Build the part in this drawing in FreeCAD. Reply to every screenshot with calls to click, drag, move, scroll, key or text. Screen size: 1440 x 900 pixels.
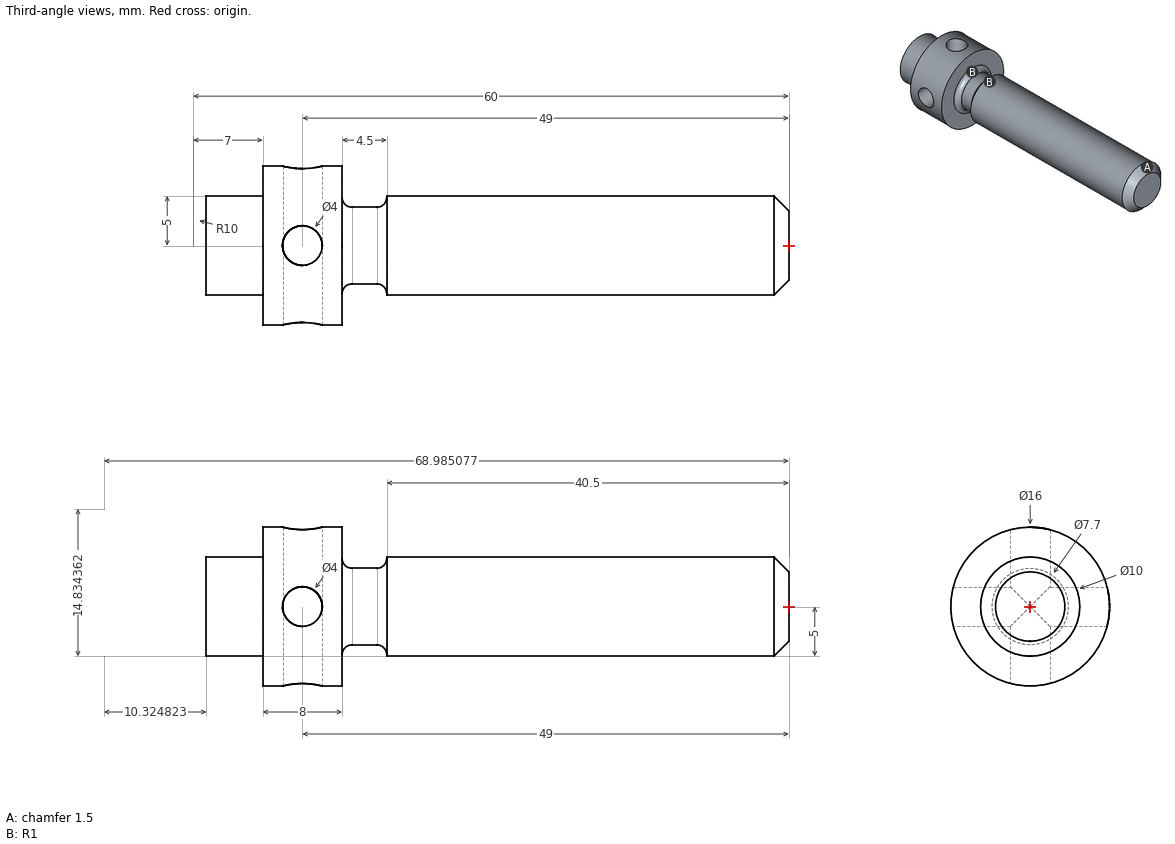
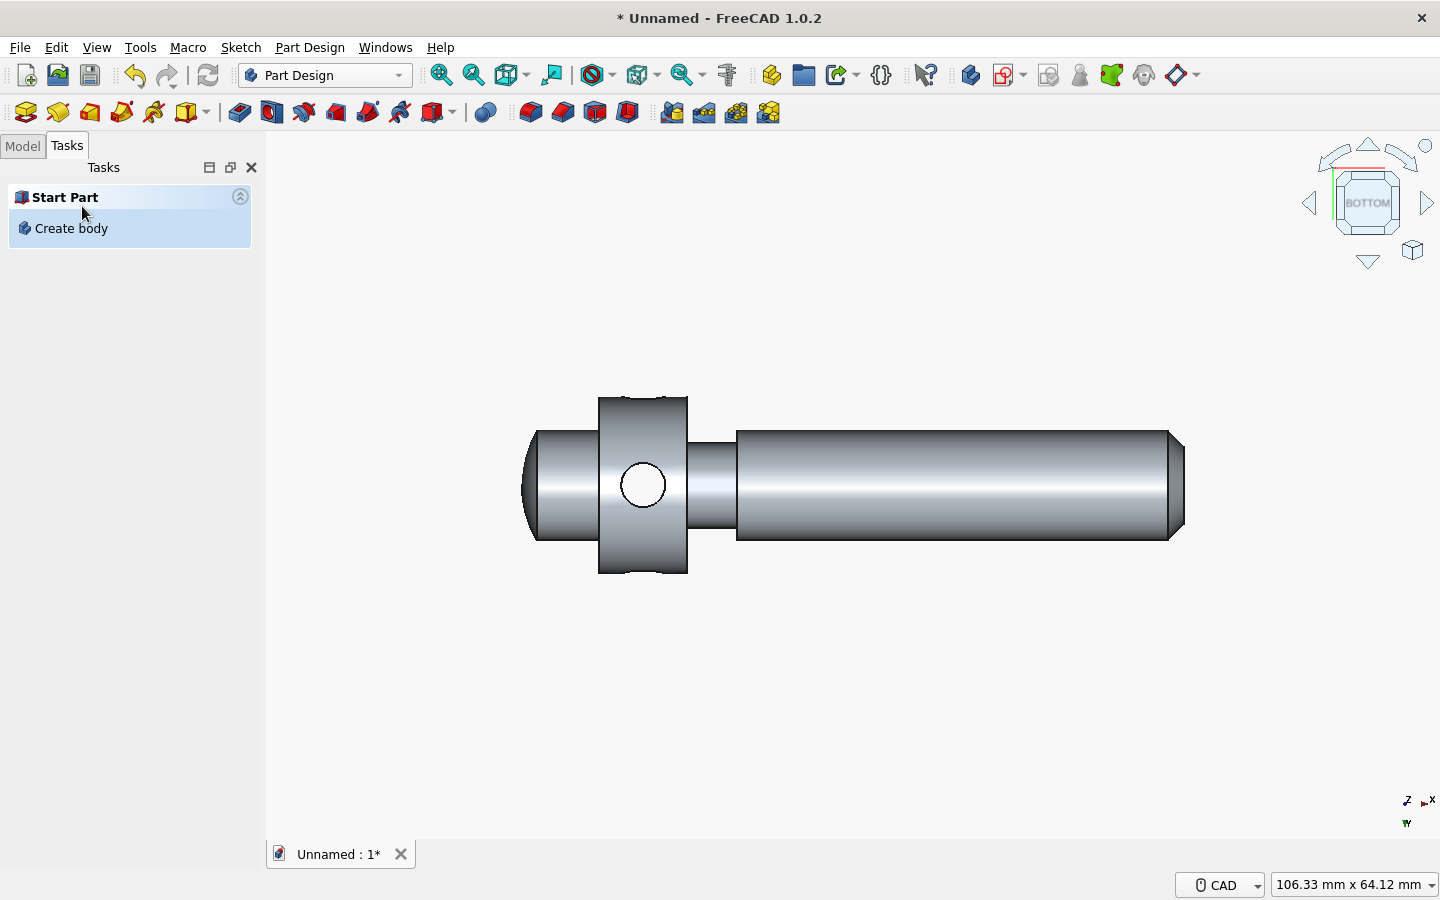
key(4)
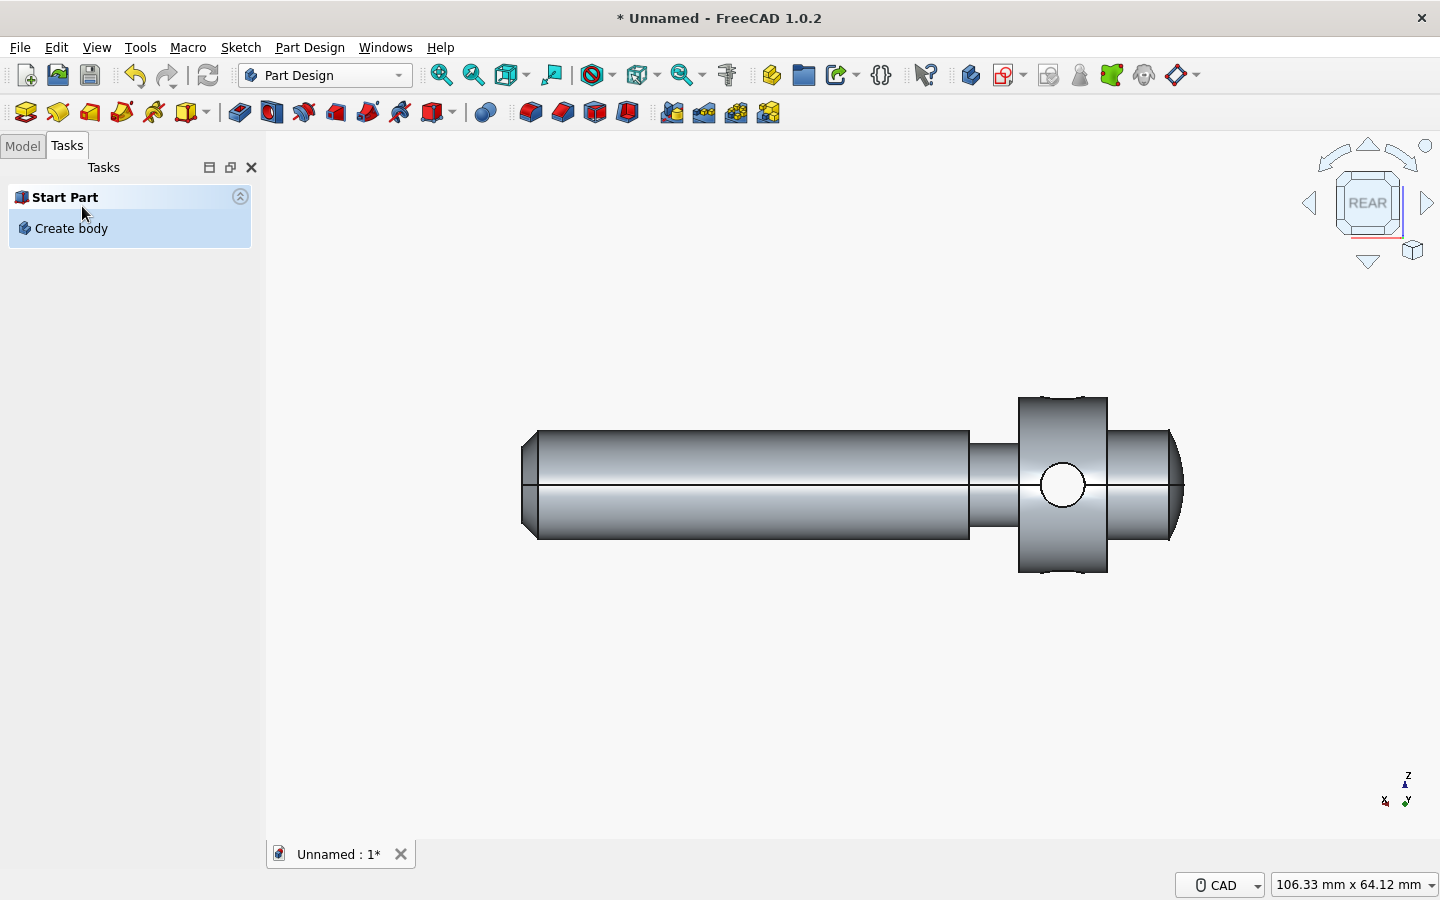
key(6)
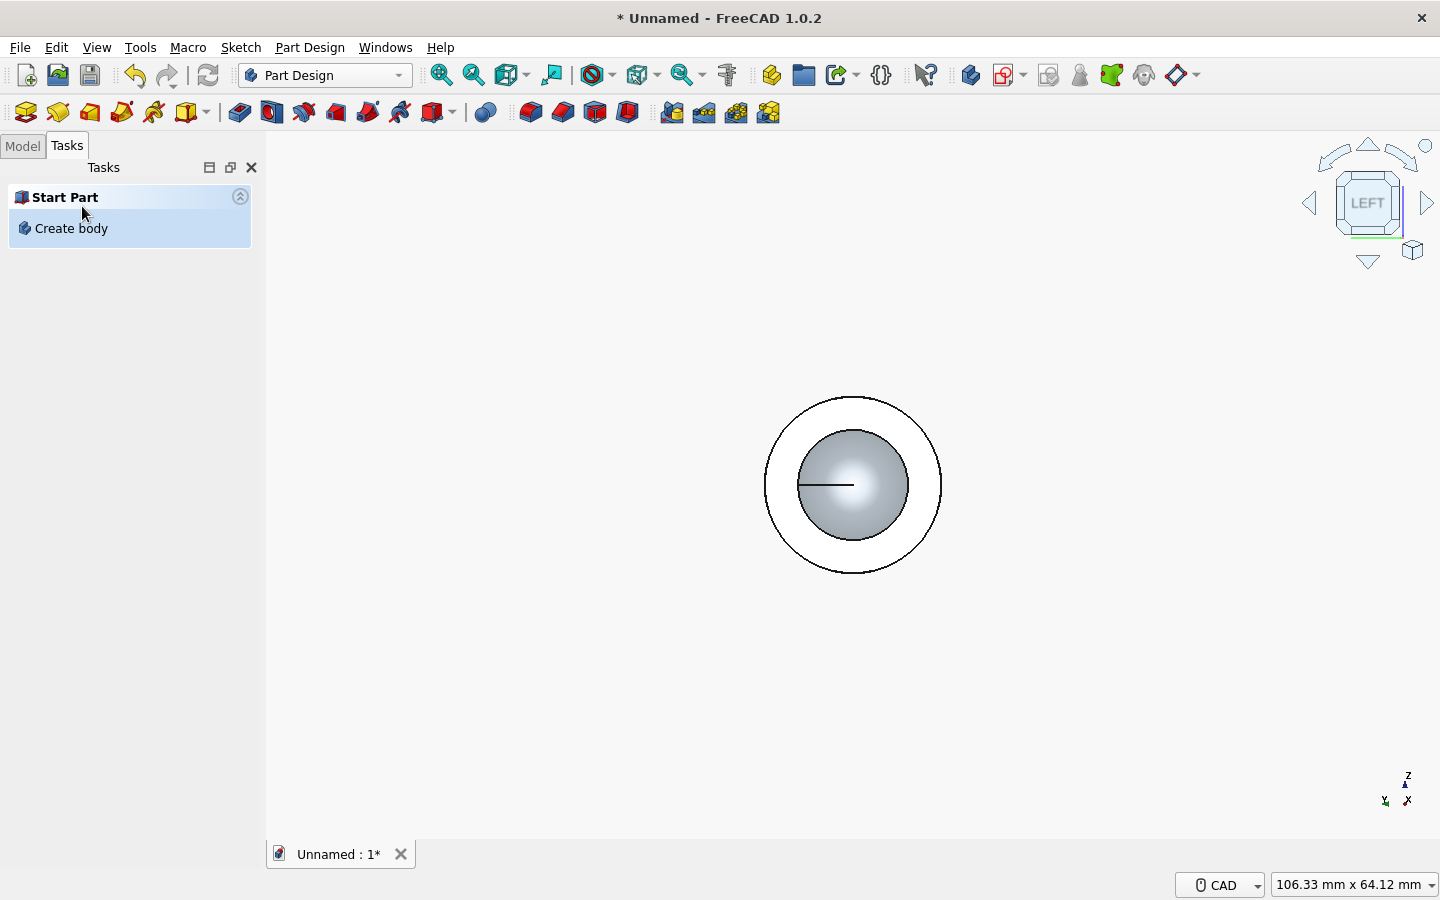
click(442, 76)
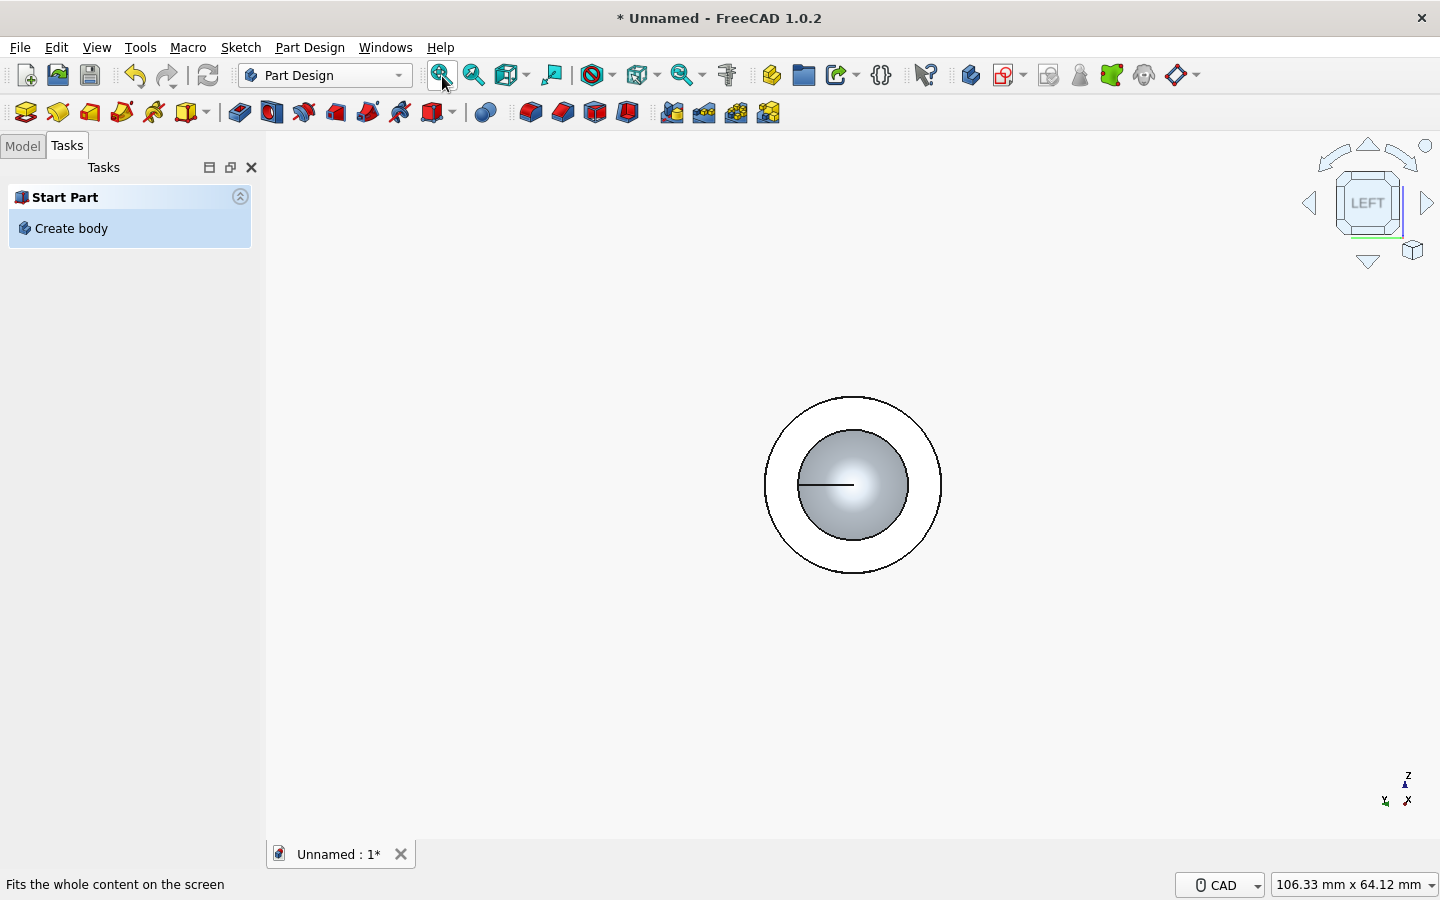
key(v)
key(3)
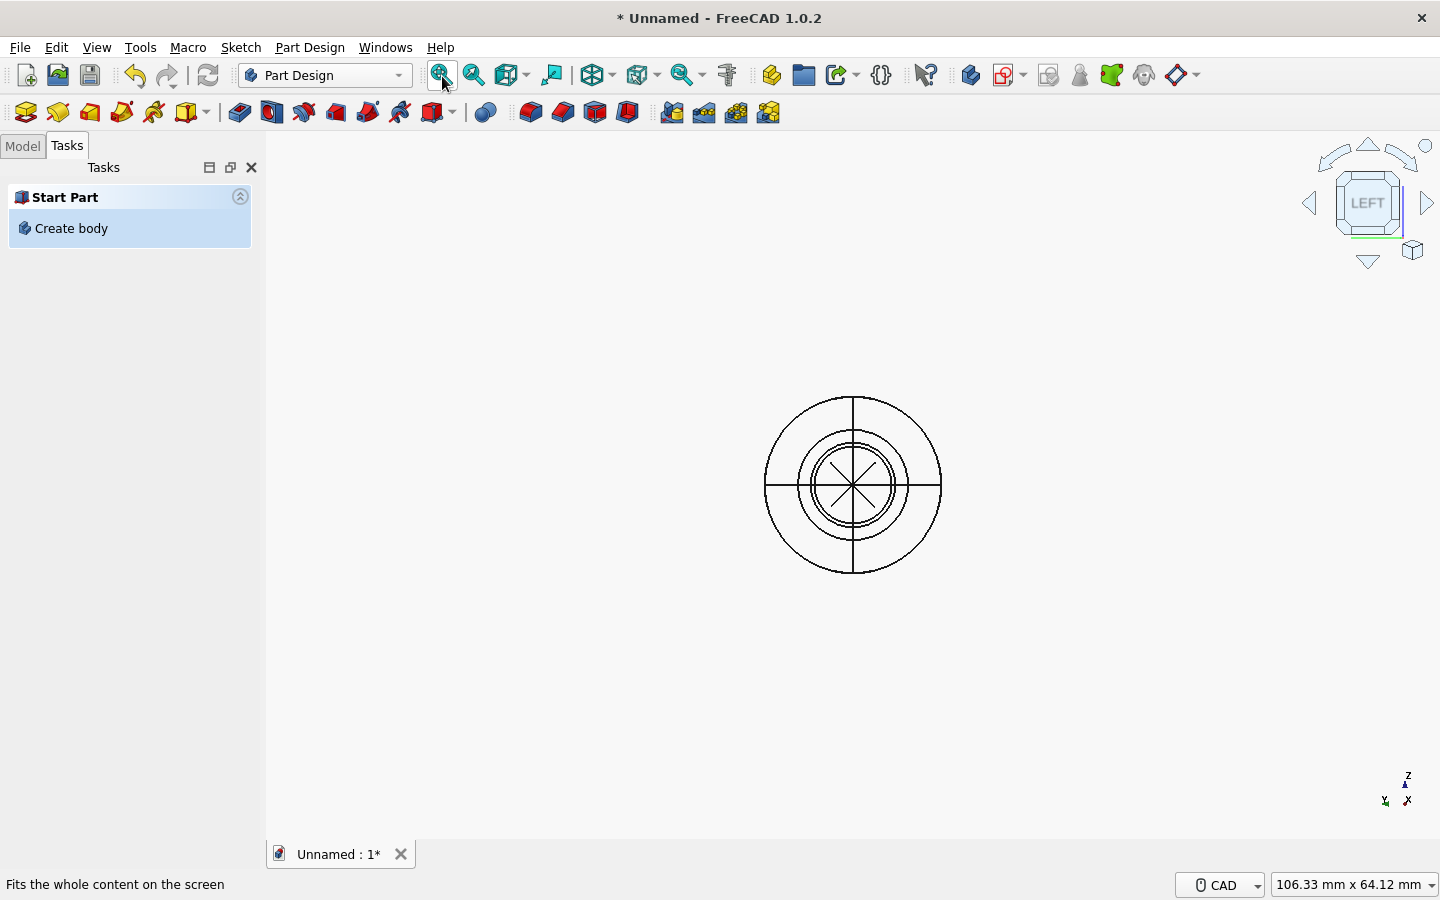
key(0)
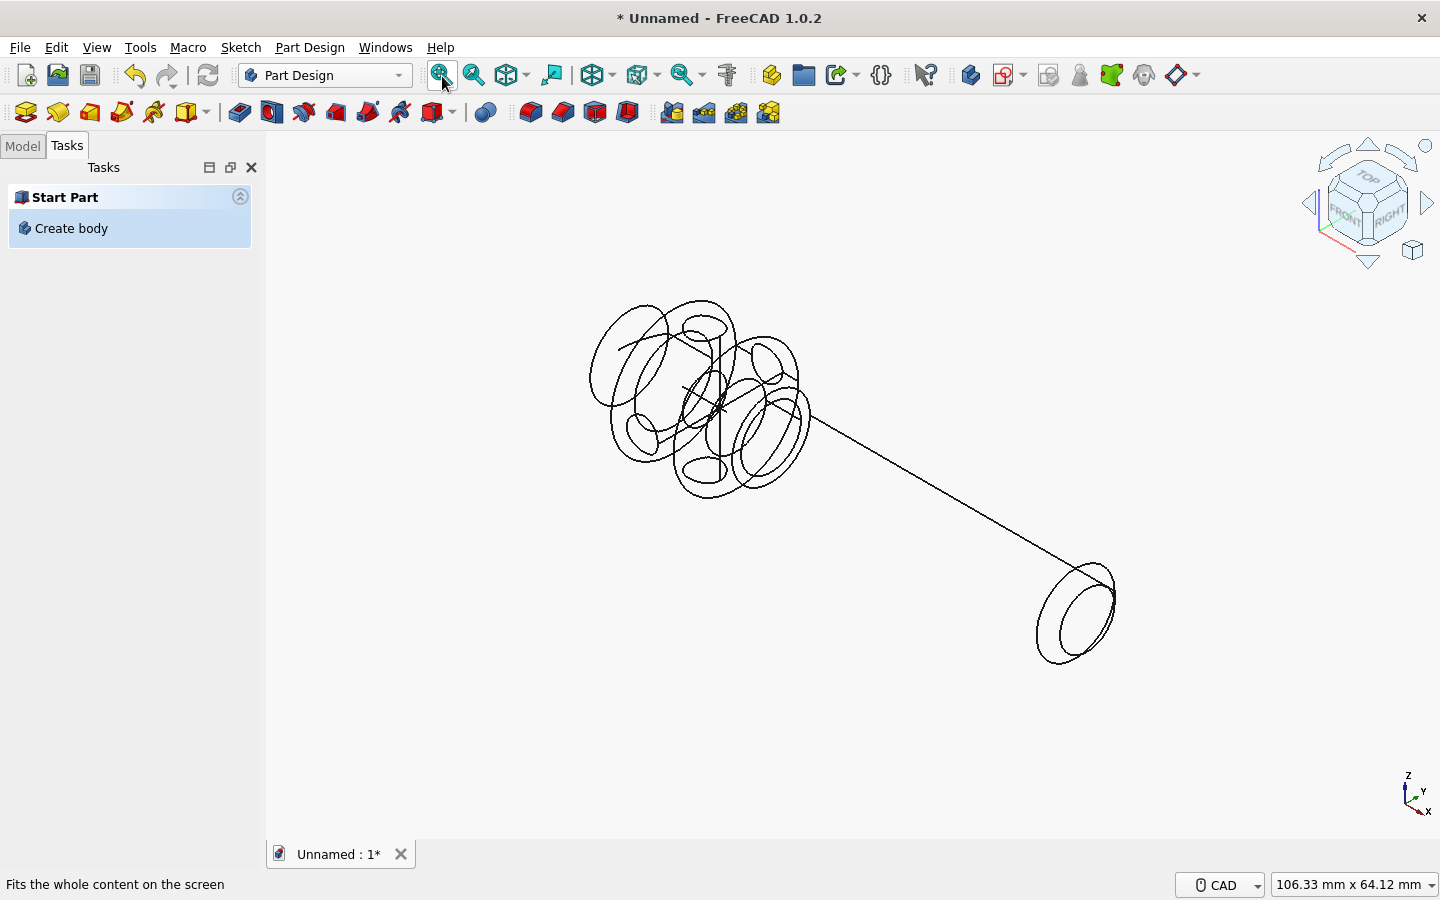
click(741, 454)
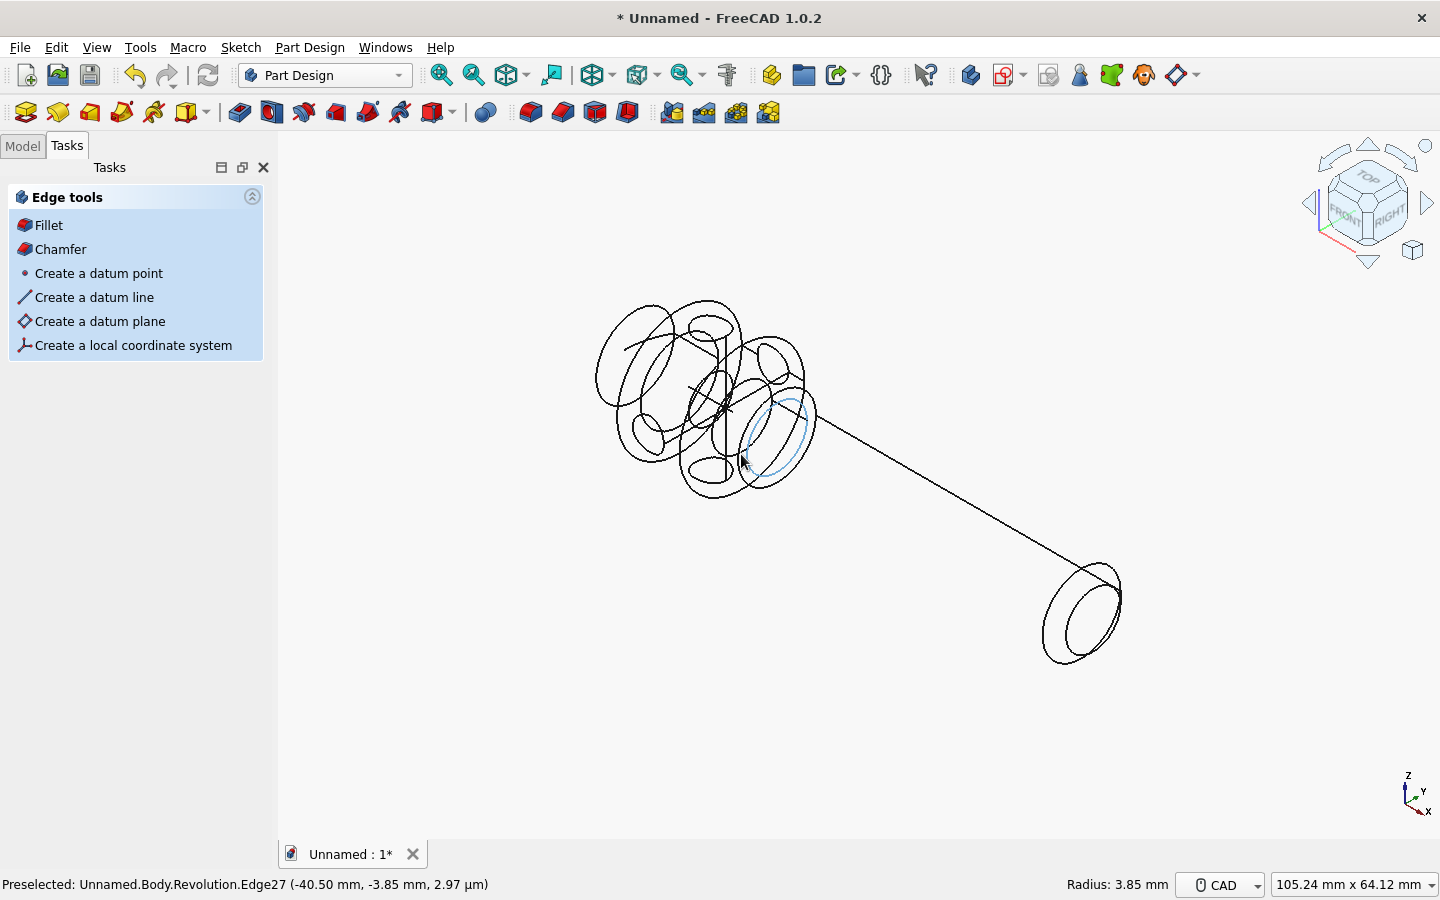
click(712, 434, ctrl)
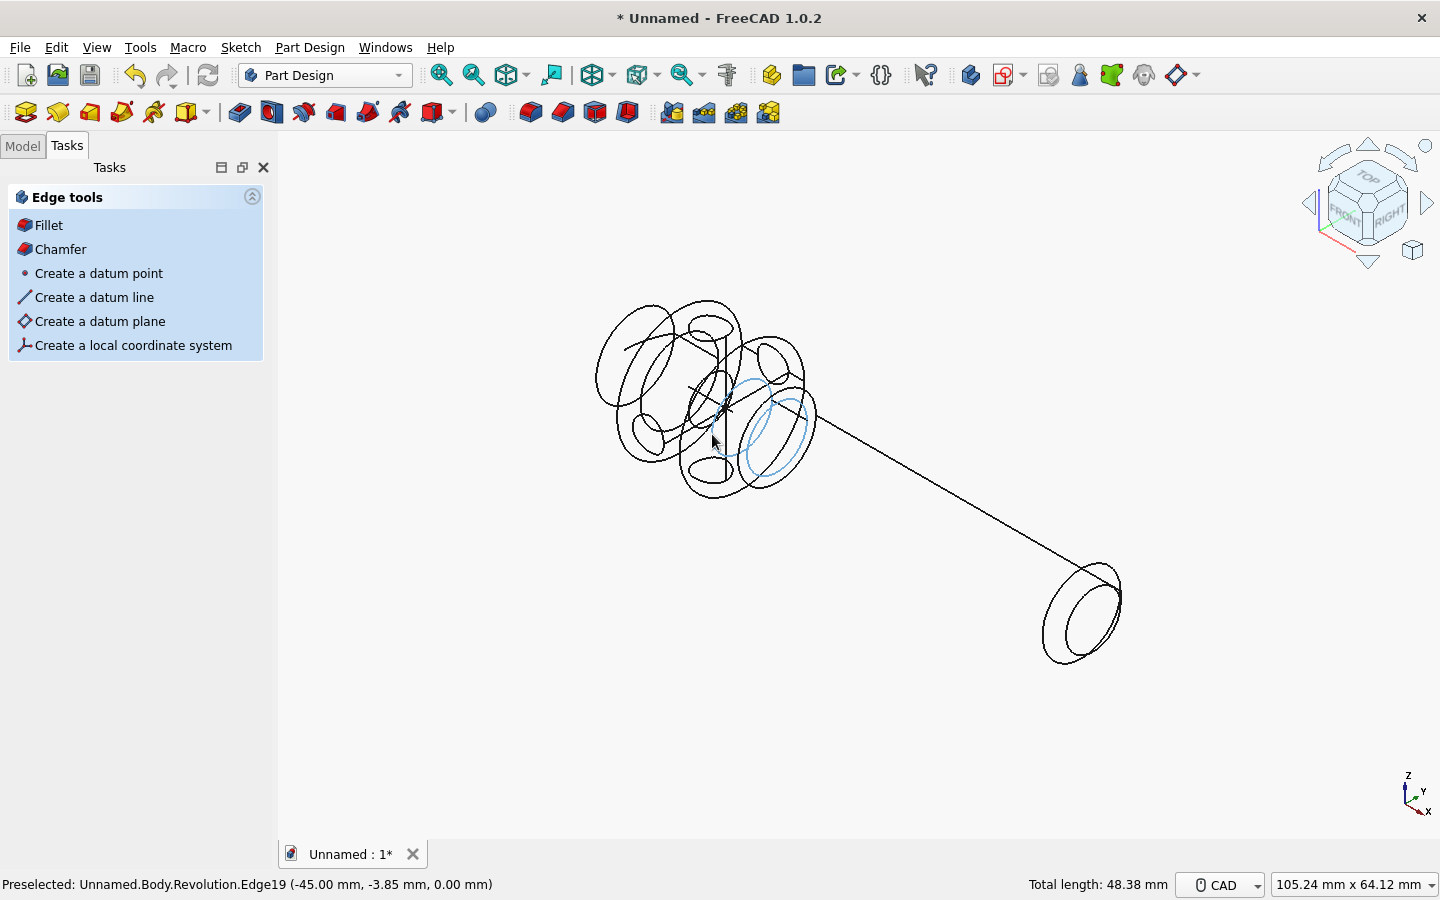
key(v)
key(1)